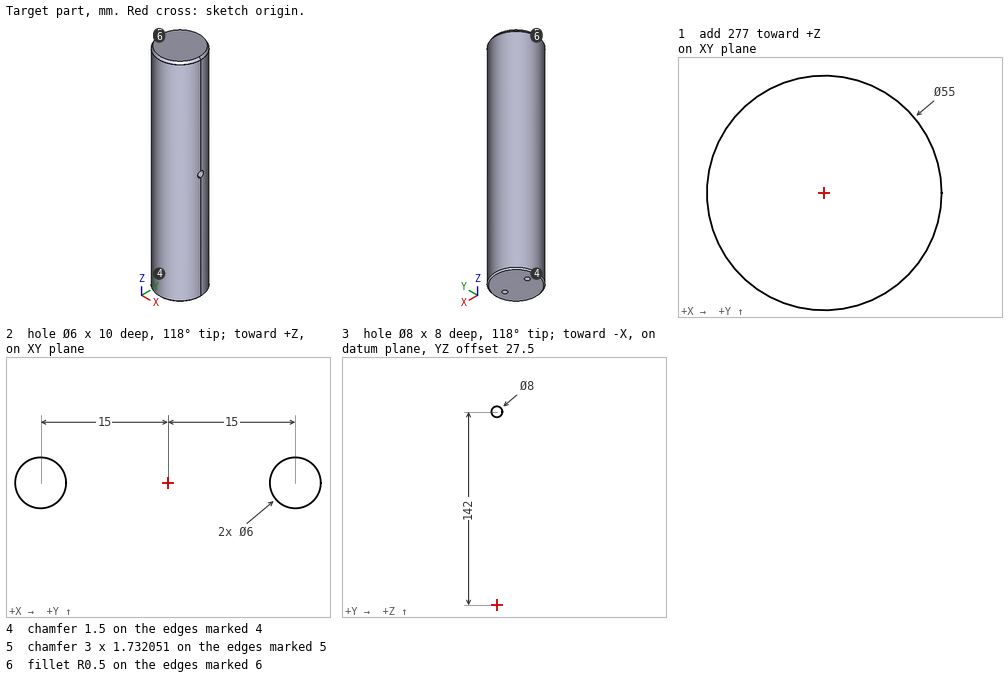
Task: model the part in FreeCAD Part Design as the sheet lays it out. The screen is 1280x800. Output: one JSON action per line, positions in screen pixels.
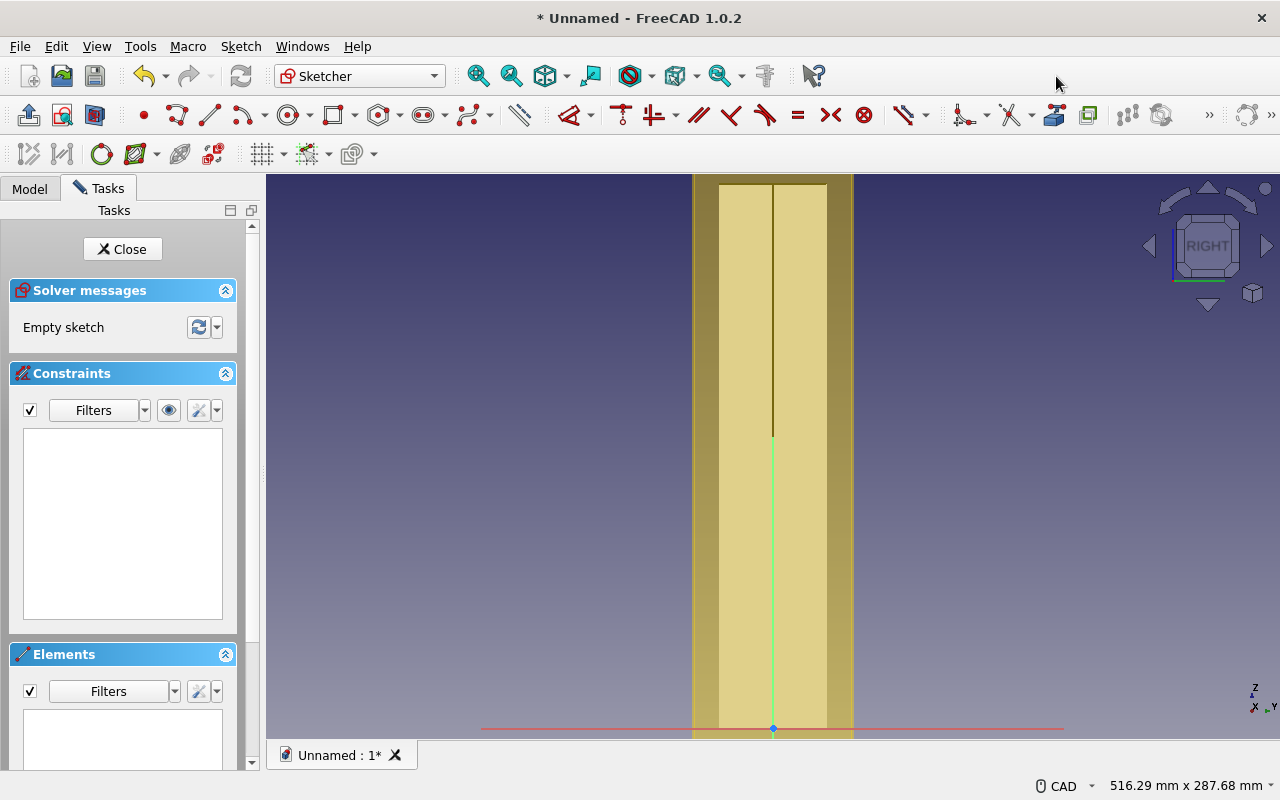
{"action": "scroll", "coordinate": [777, 449], "scroll_direction": "up", "scroll_amount": 15}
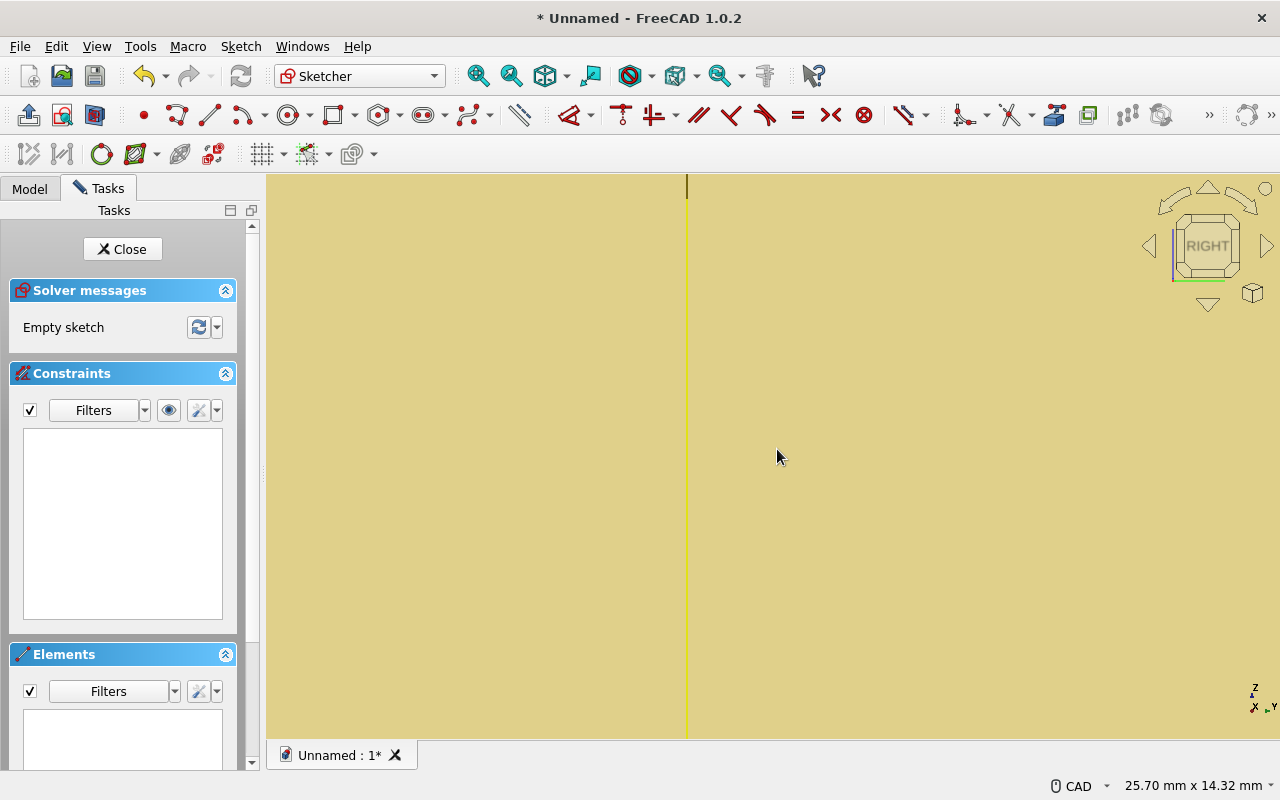
{"action": "key", "text": "g c"}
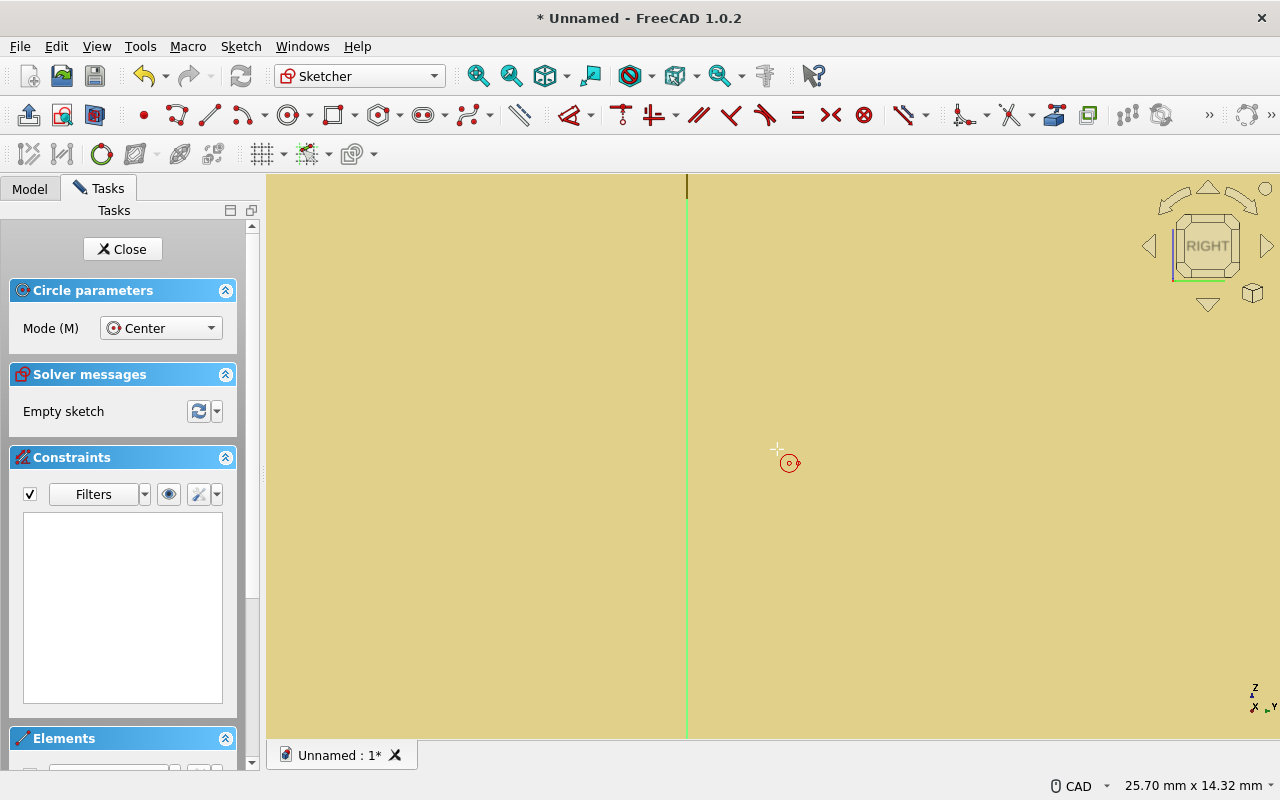
{"action": "left_click", "coordinate": [687, 452]}
{"action": "left_click", "coordinate": [799, 341]}
{"action": "key", "text": "Escape"}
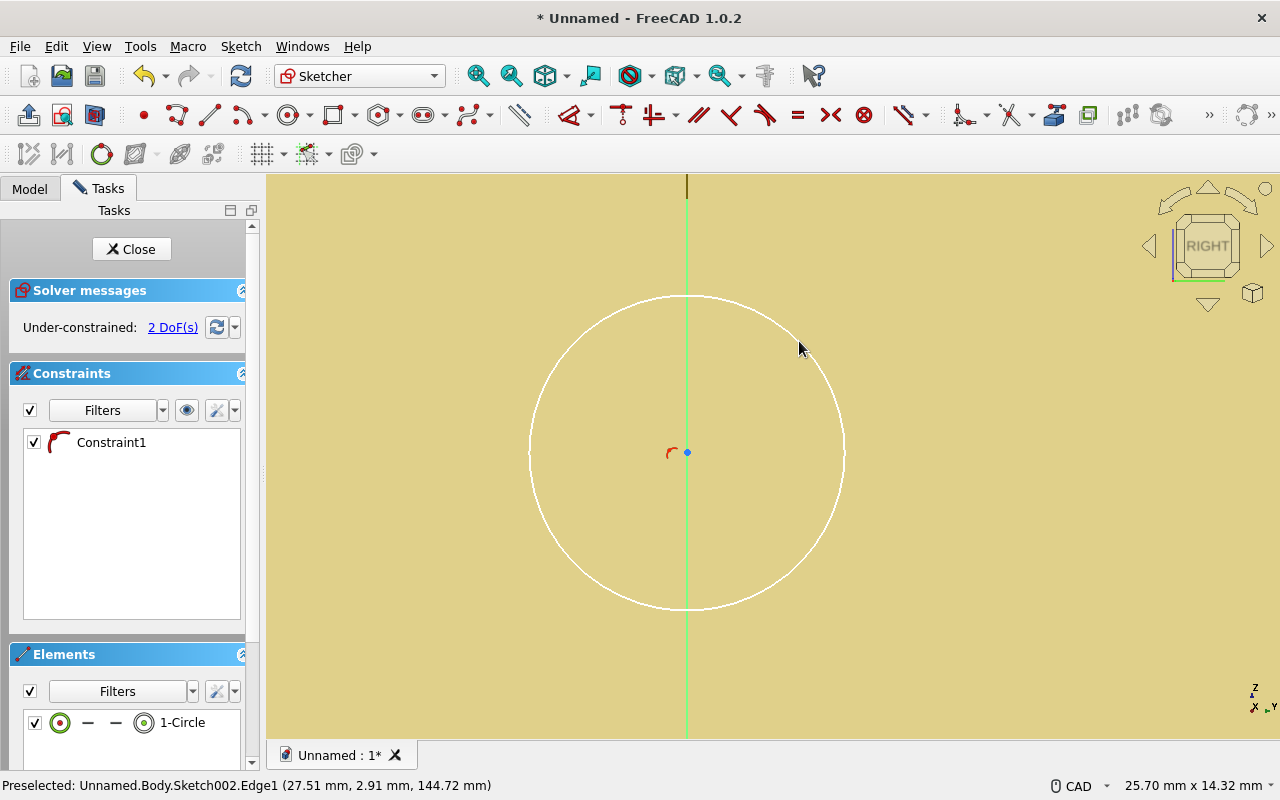
{"action": "left_click", "coordinate": [568, 116]}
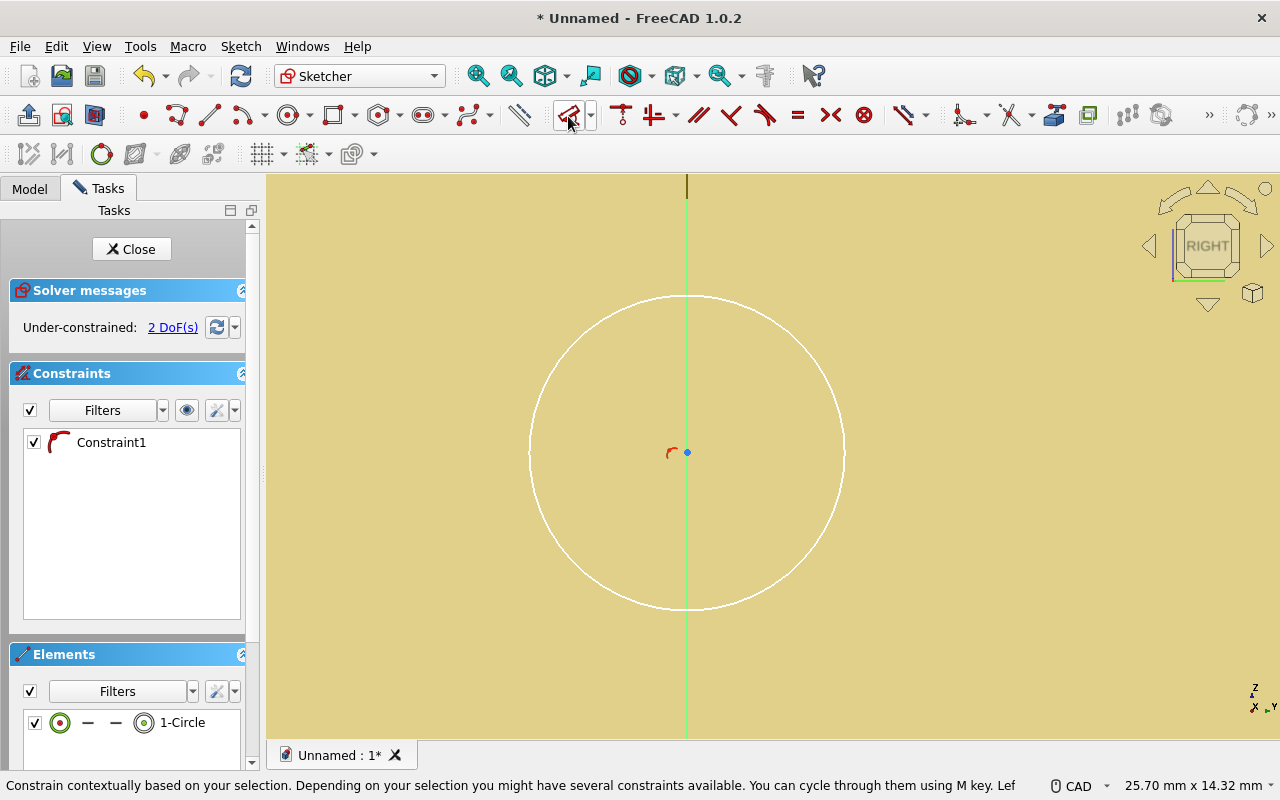
{"action": "left_click", "coordinate": [798, 341]}
{"action": "left_click", "coordinate": [821, 318]}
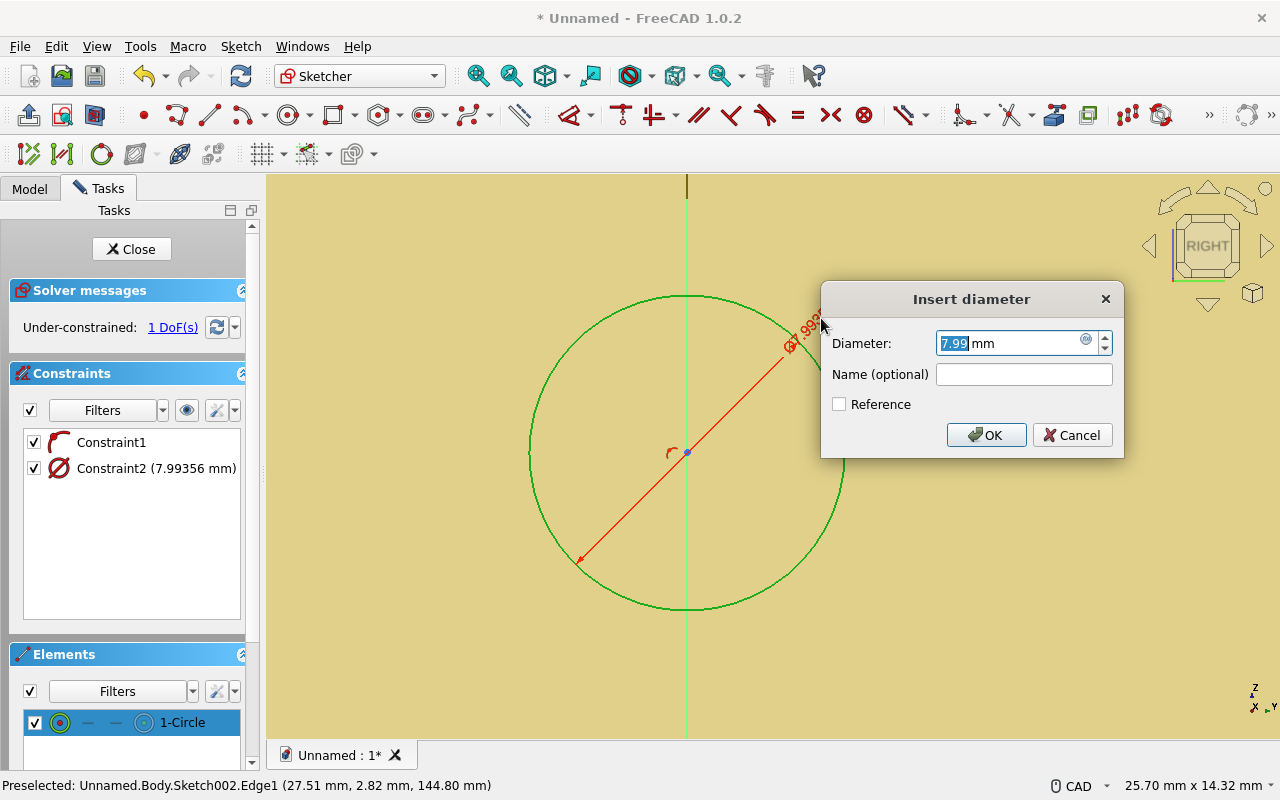
{"action": "type", "text": "8"}
{"action": "key", "text": "Return"}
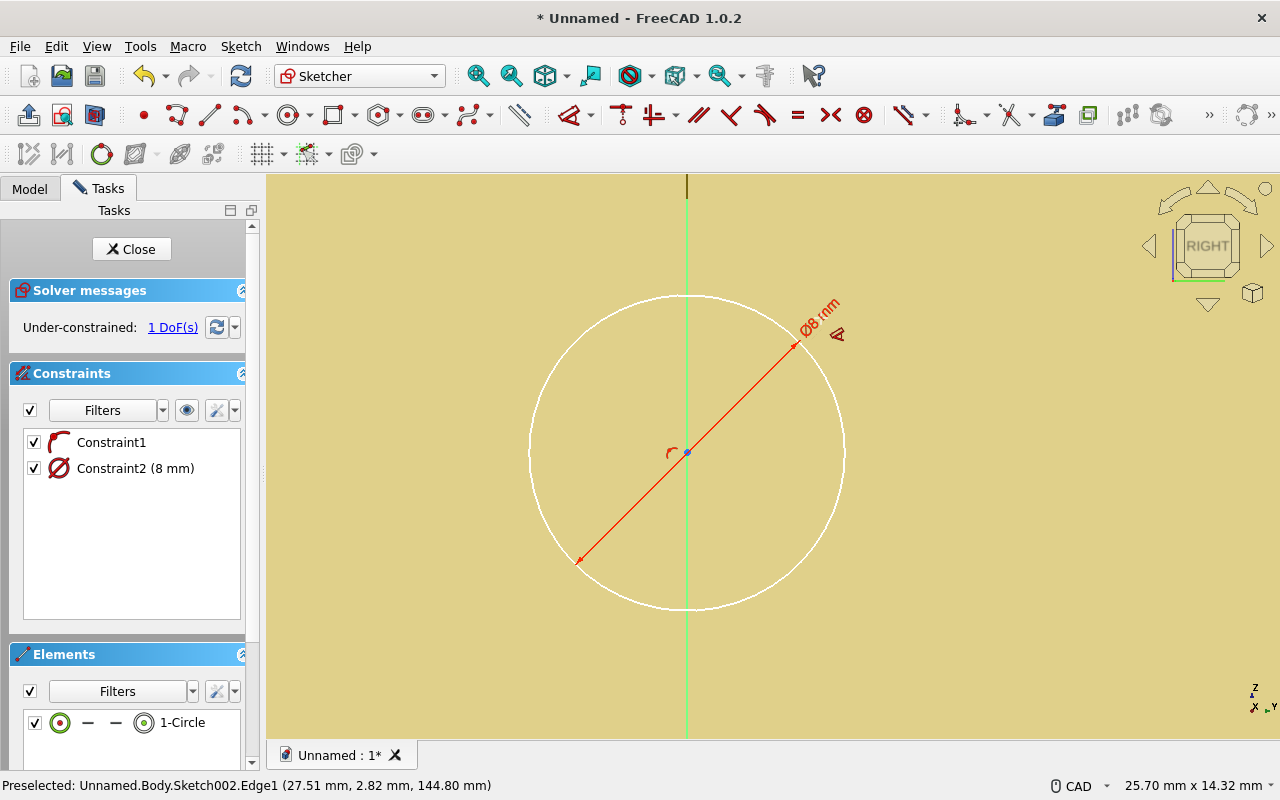
{"action": "left_click", "coordinate": [687, 453]}
{"action": "left_click", "coordinate": [721, 582]}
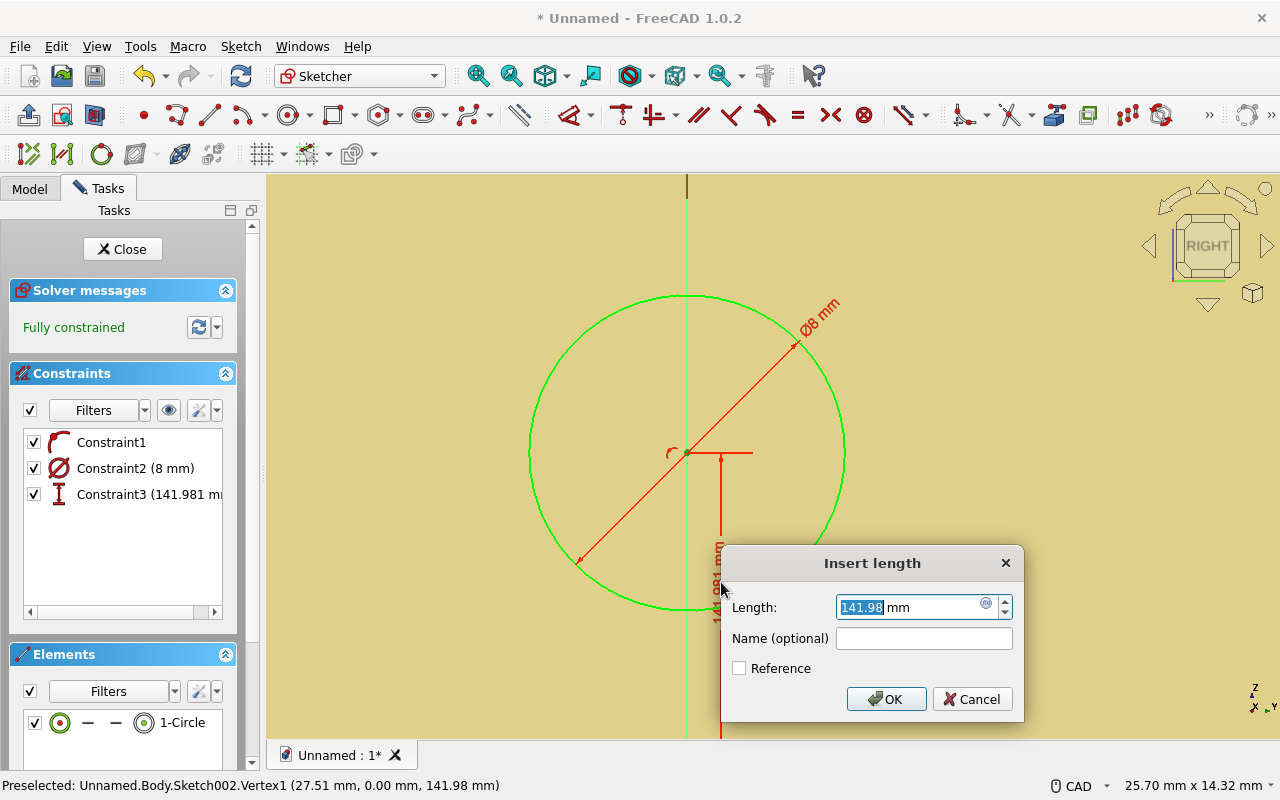
{"action": "type", "text": "142"}
{"action": "key", "text": "Return"}
{"action": "key", "text": "Escape"}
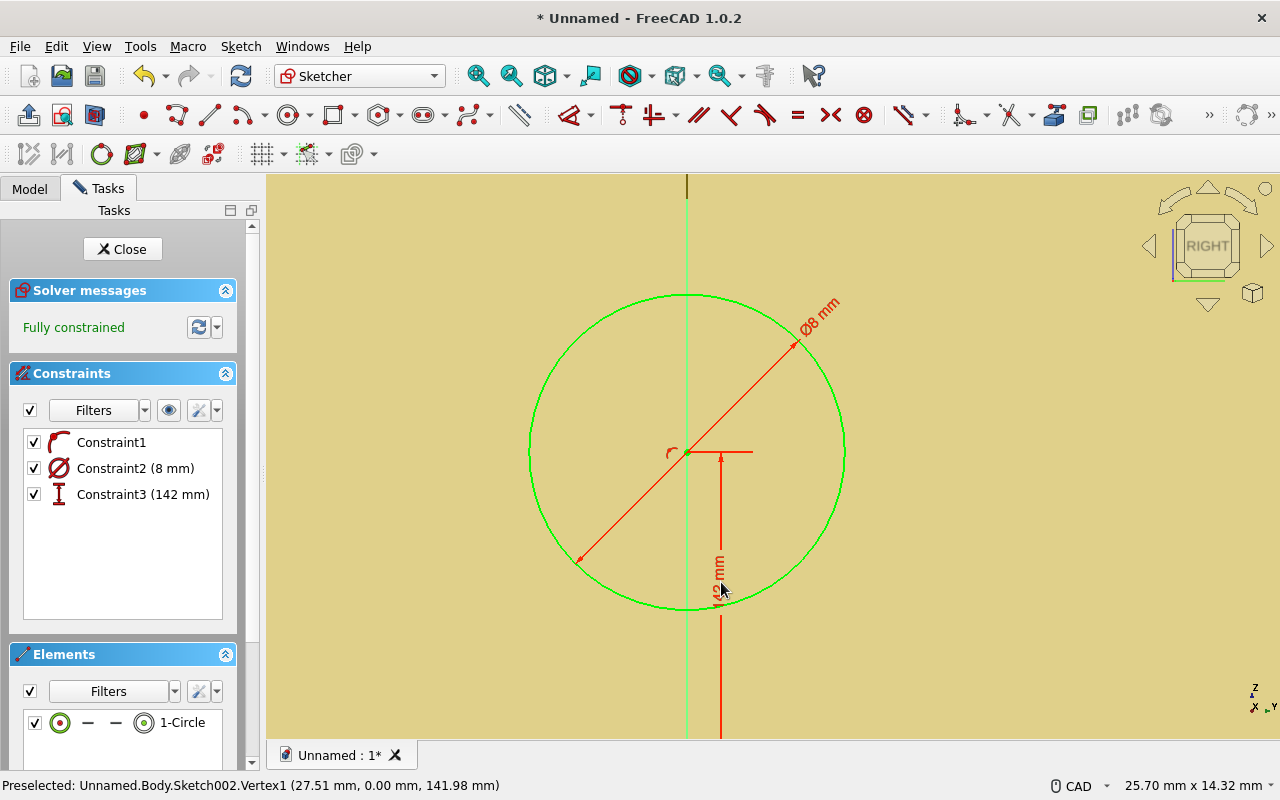
{"action": "left_click", "coordinate": [123, 249]}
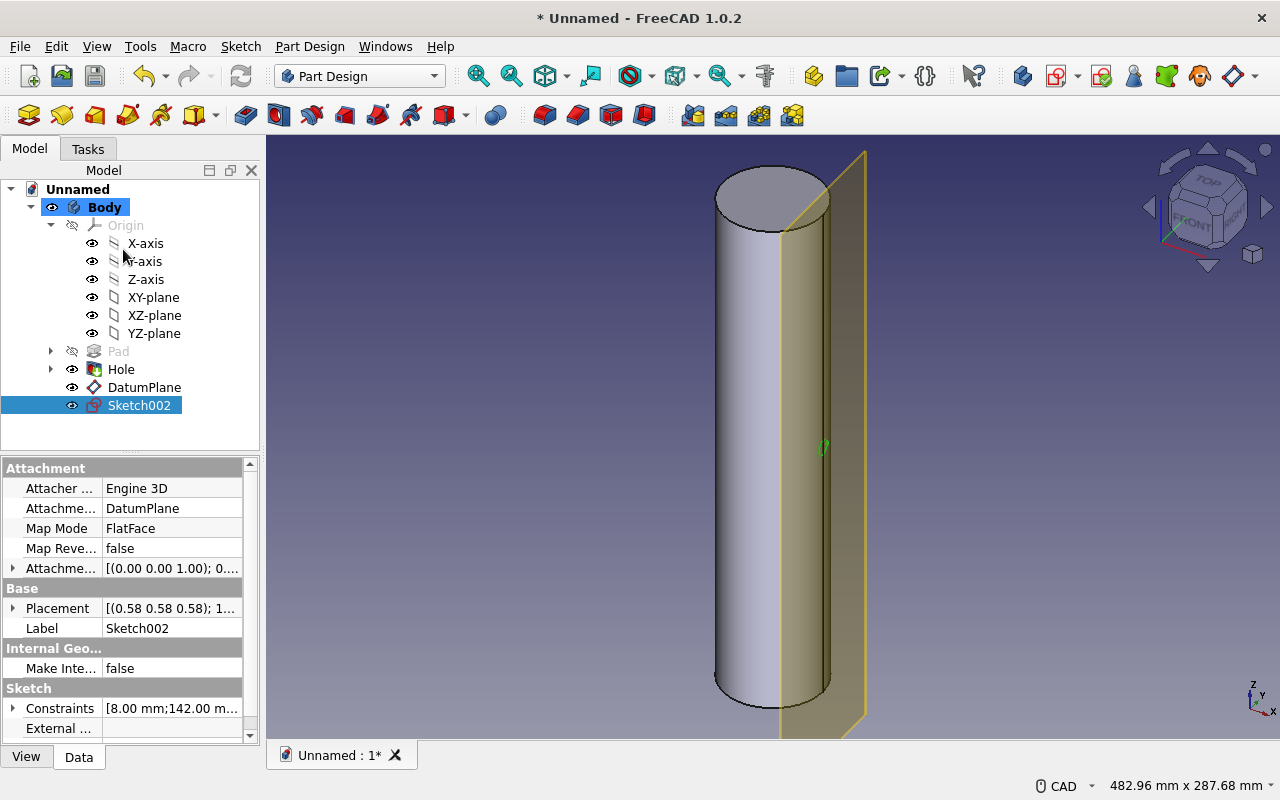
{"action": "left_click", "coordinate": [279, 116]}